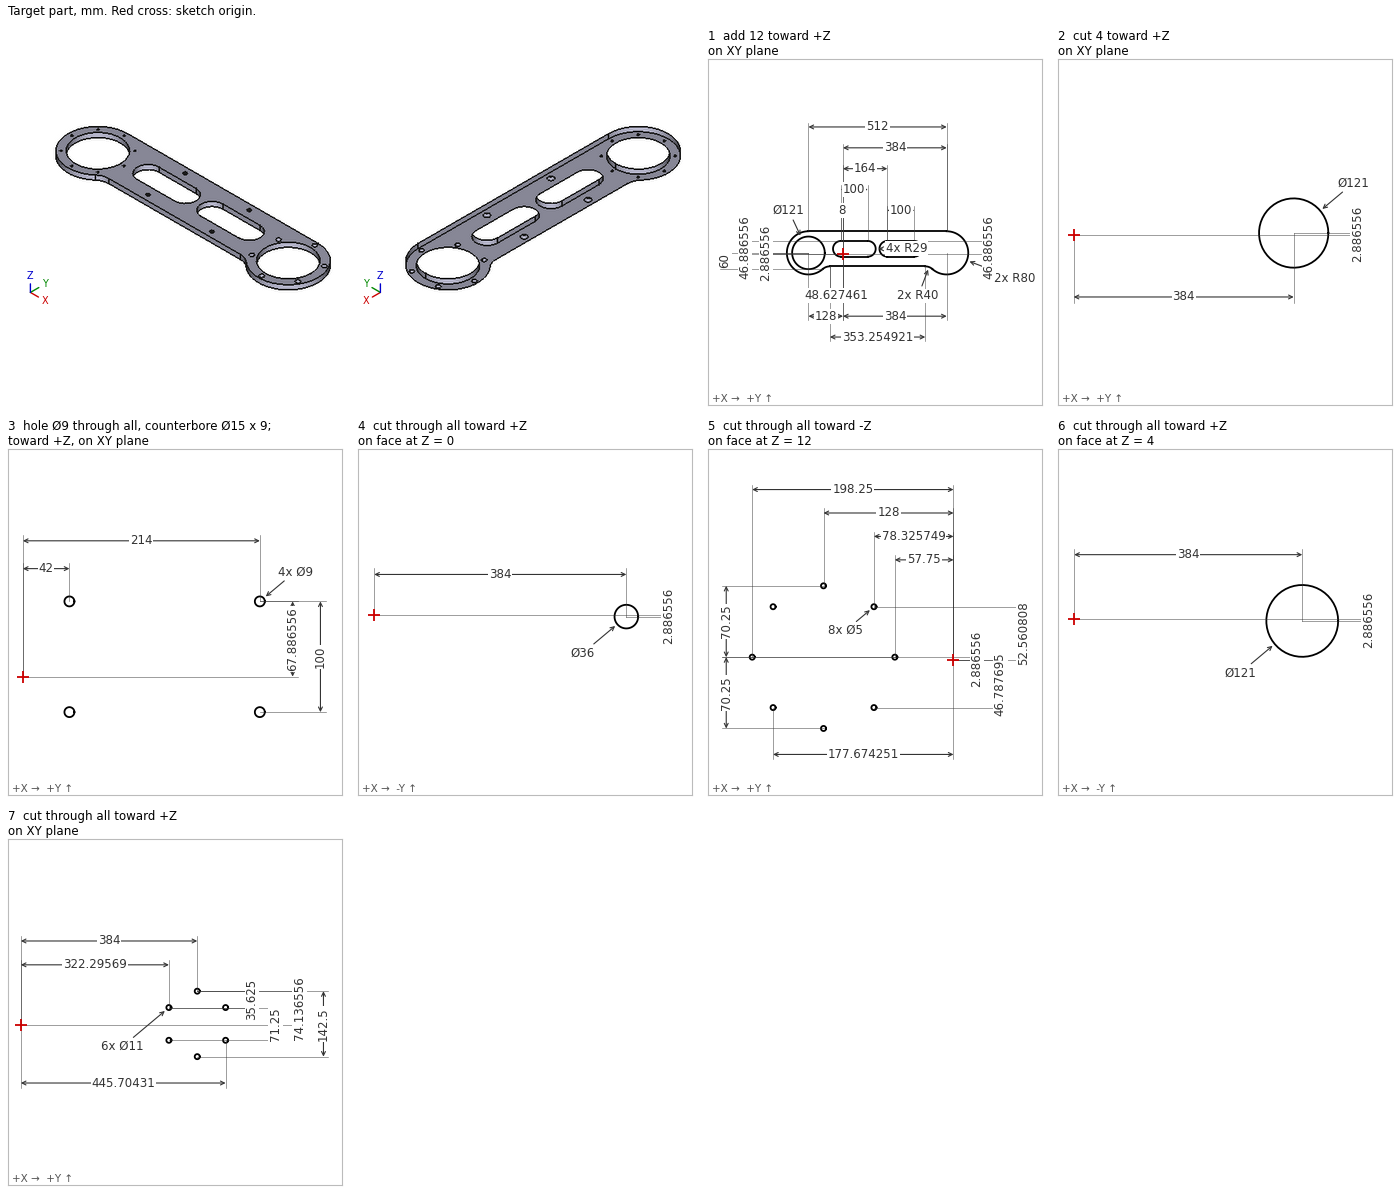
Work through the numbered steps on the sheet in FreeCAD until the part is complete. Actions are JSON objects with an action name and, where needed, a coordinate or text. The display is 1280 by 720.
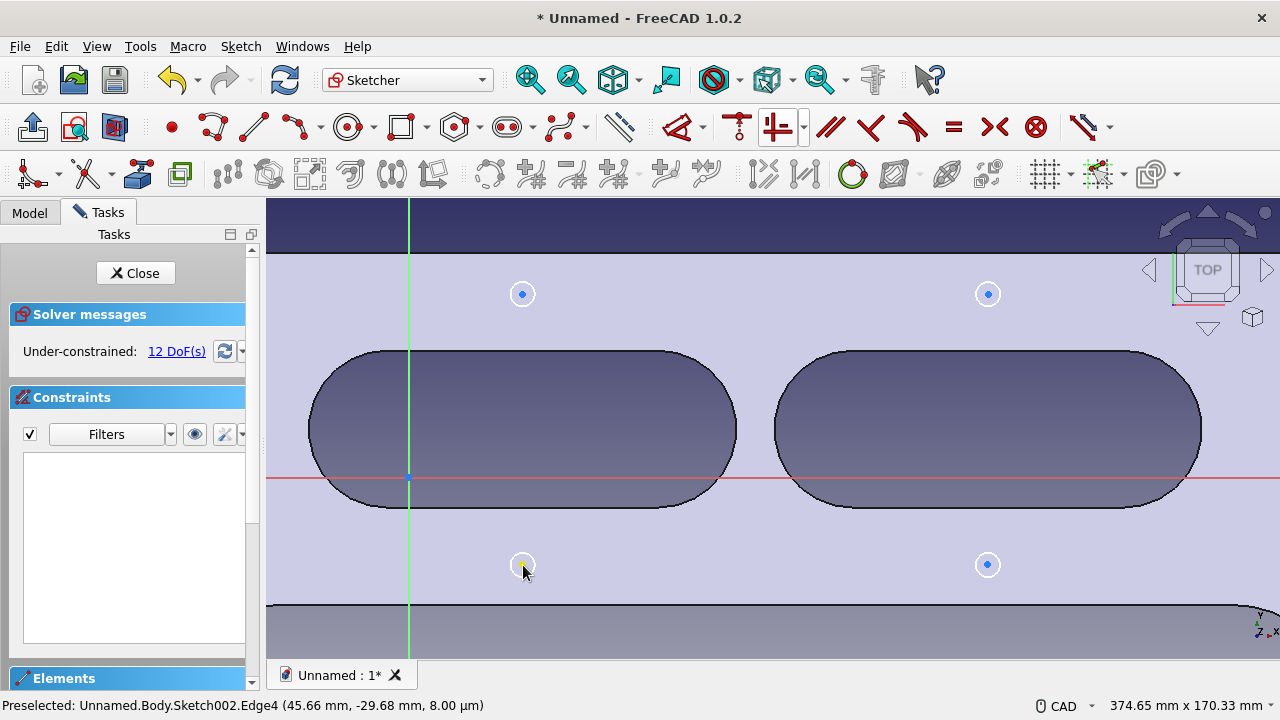
{"action": "left_click", "coordinate": [997, 286]}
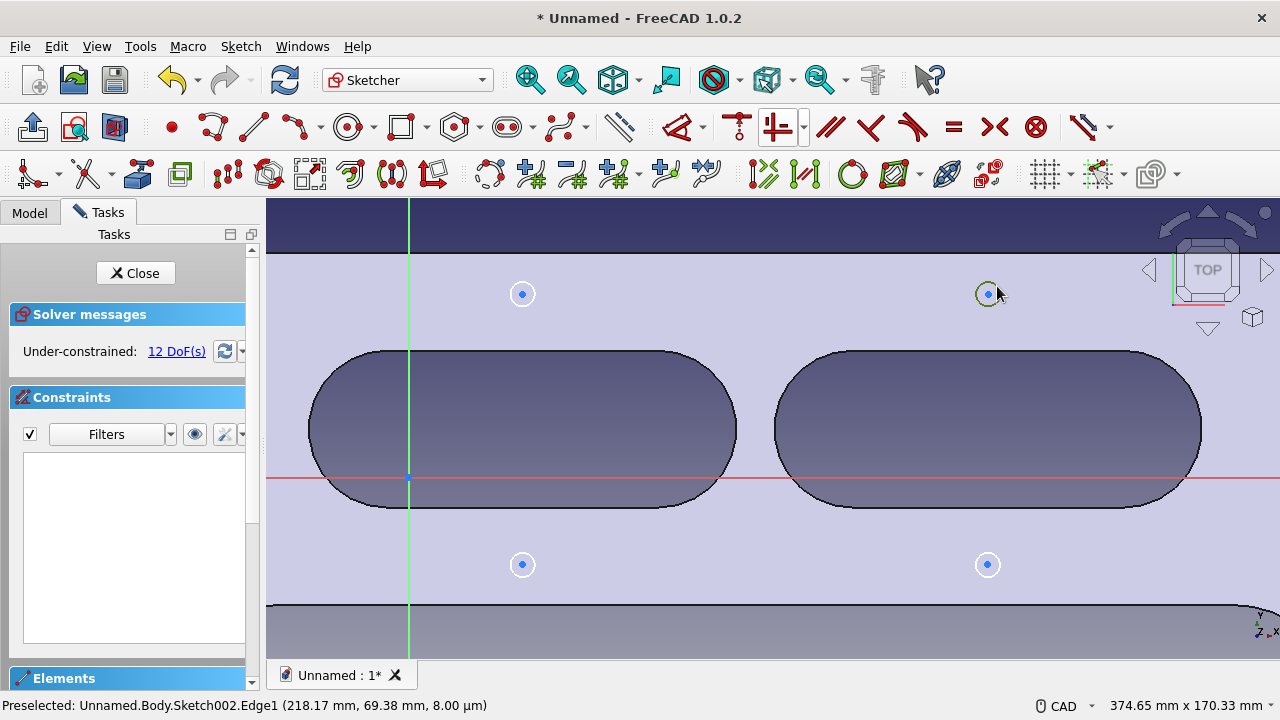
{"action": "left_click", "coordinate": [996, 556]}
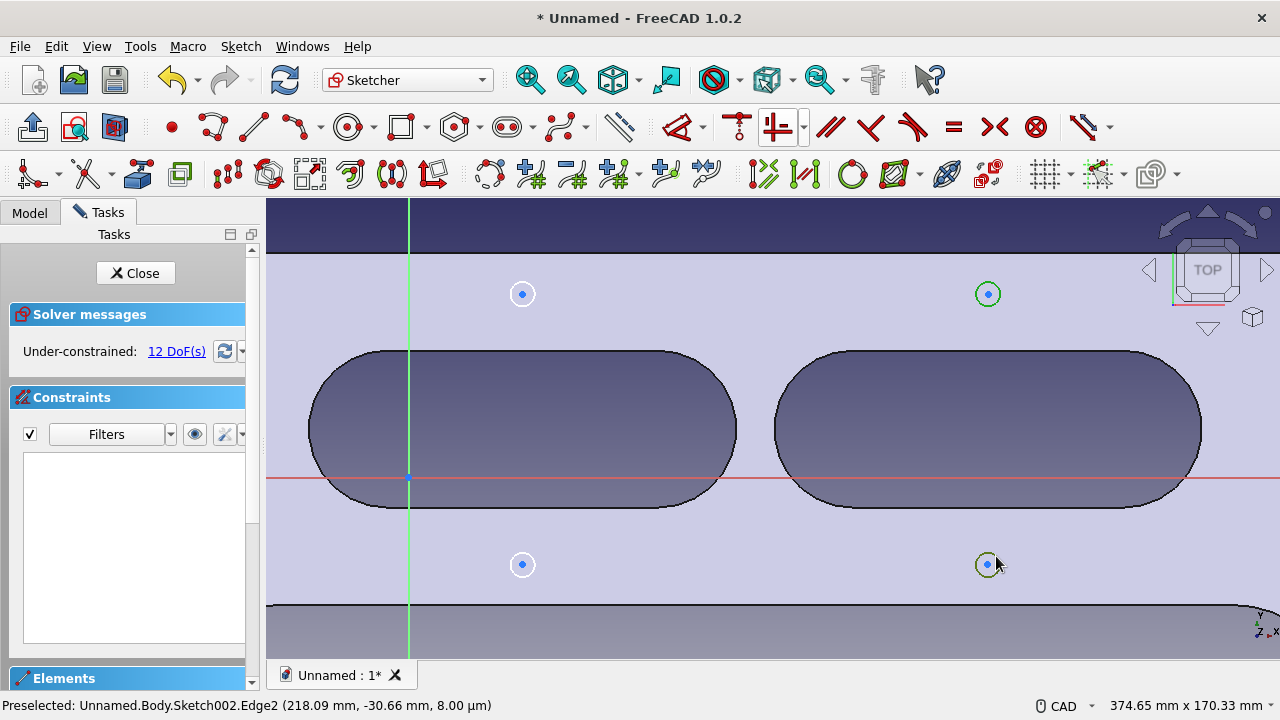
{"action": "left_click", "coordinate": [531, 286]}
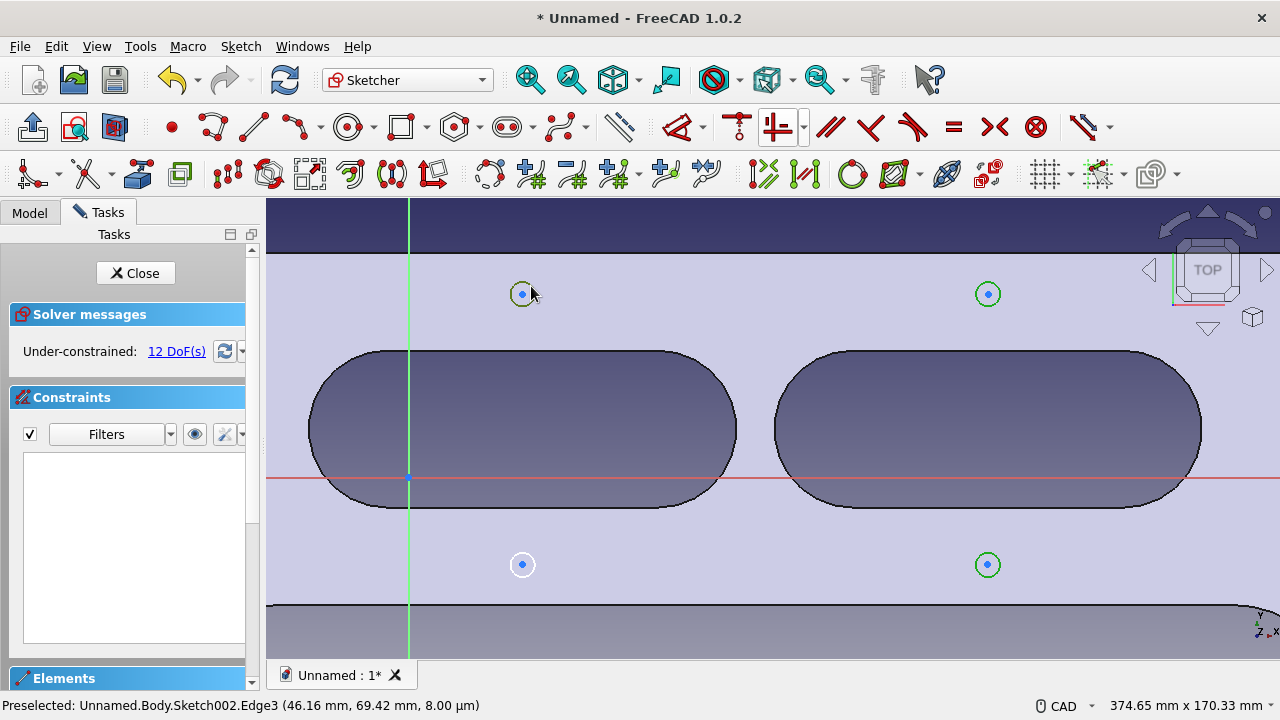
{"action": "left_click", "coordinate": [531, 556]}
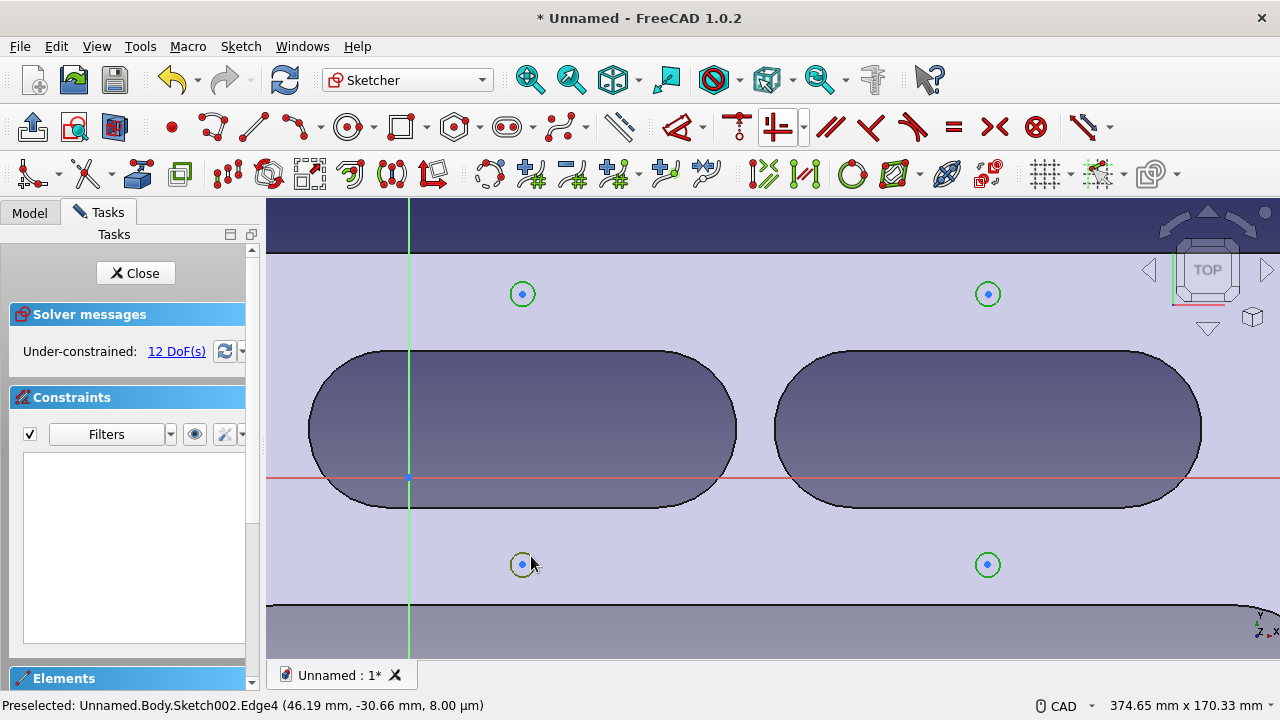
{"action": "left_click", "coordinate": [954, 128]}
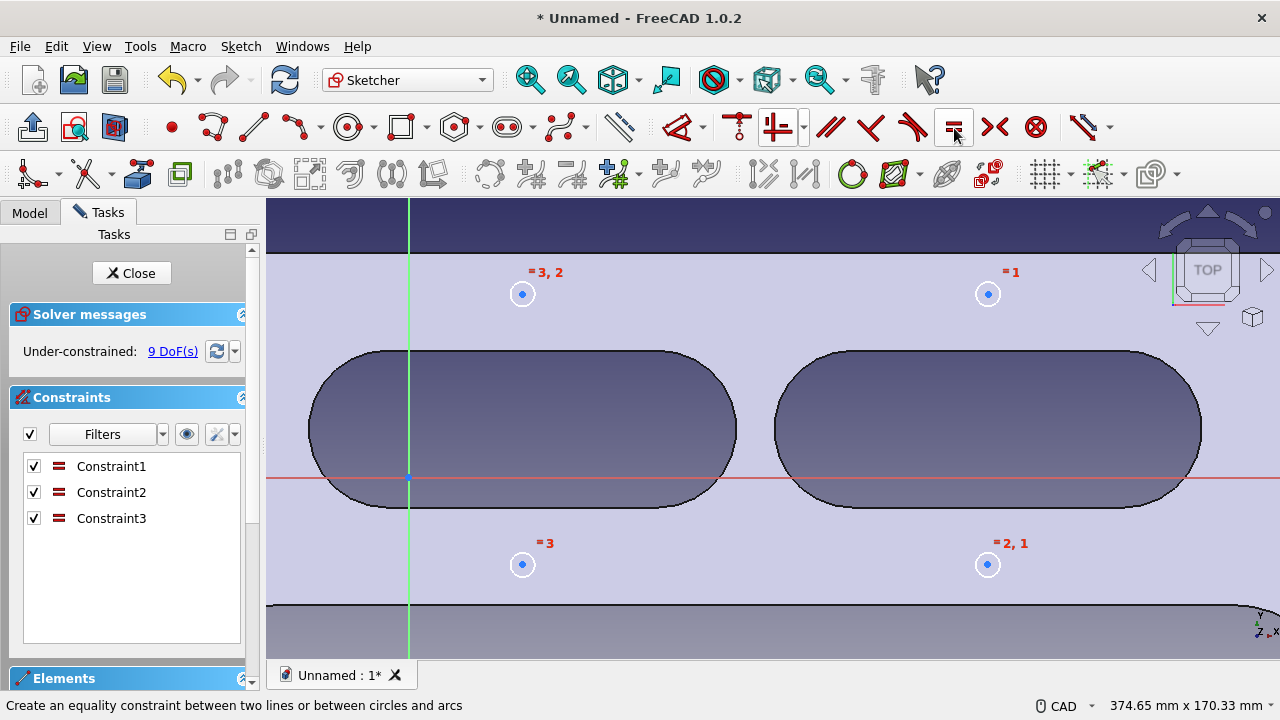
{"action": "left_click", "coordinate": [988, 294]}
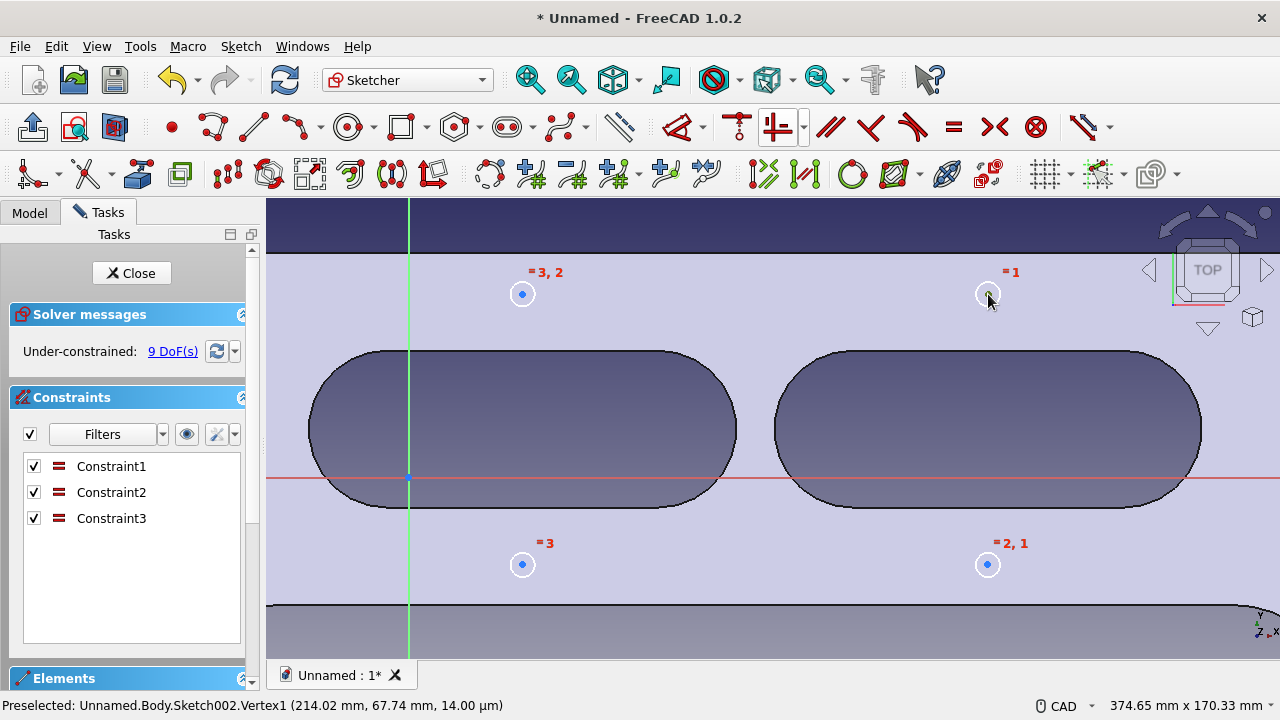
{"action": "left_click", "coordinate": [988, 565]}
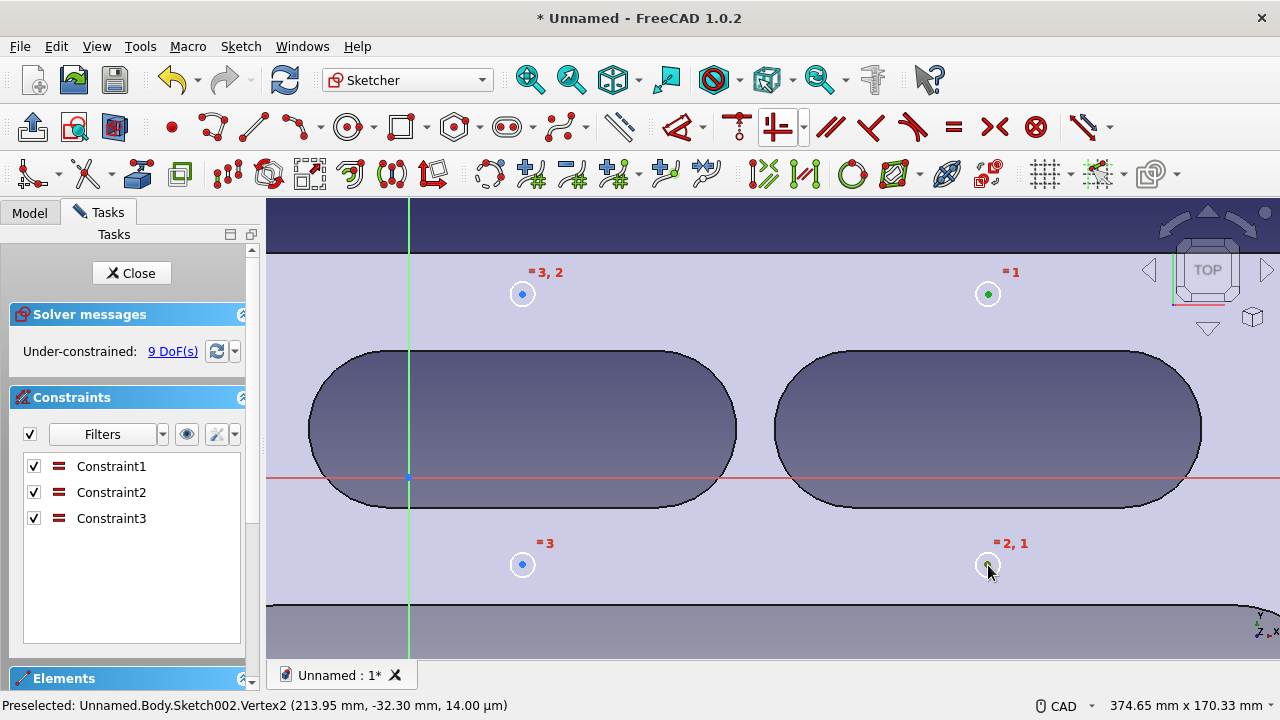
{"action": "key", "text": "v"}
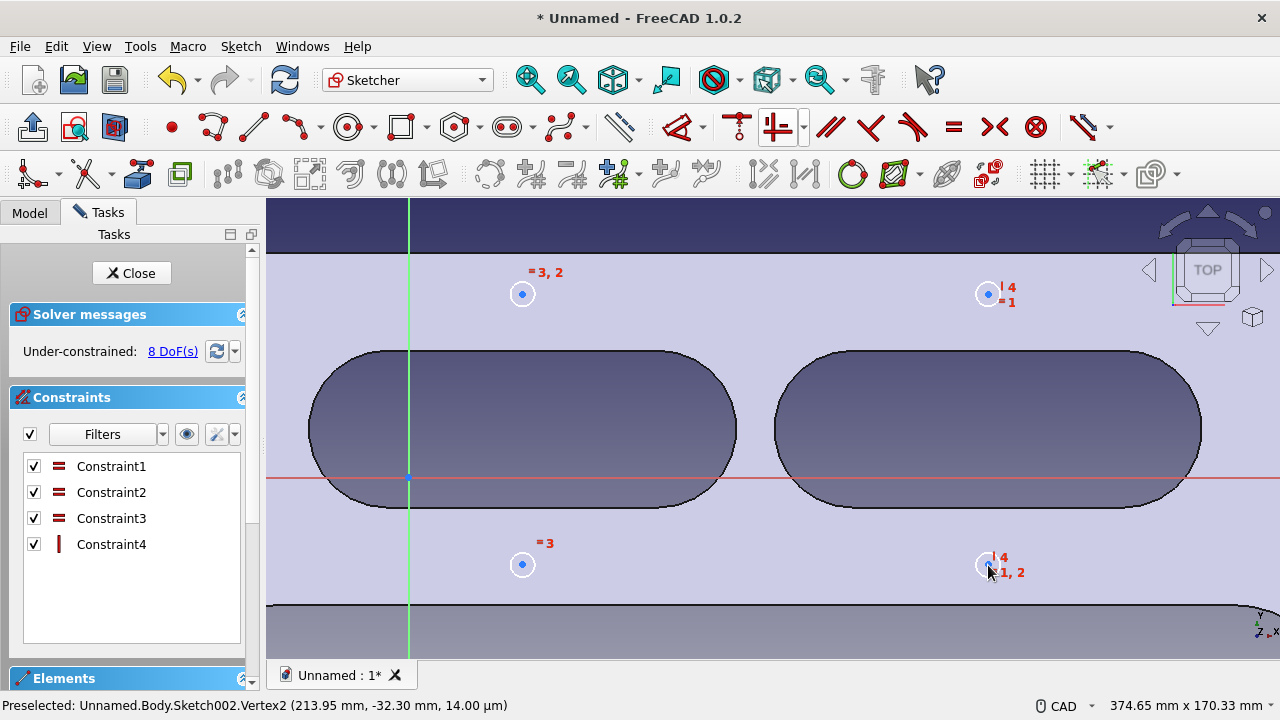
{"action": "left_click", "coordinate": [988, 294]}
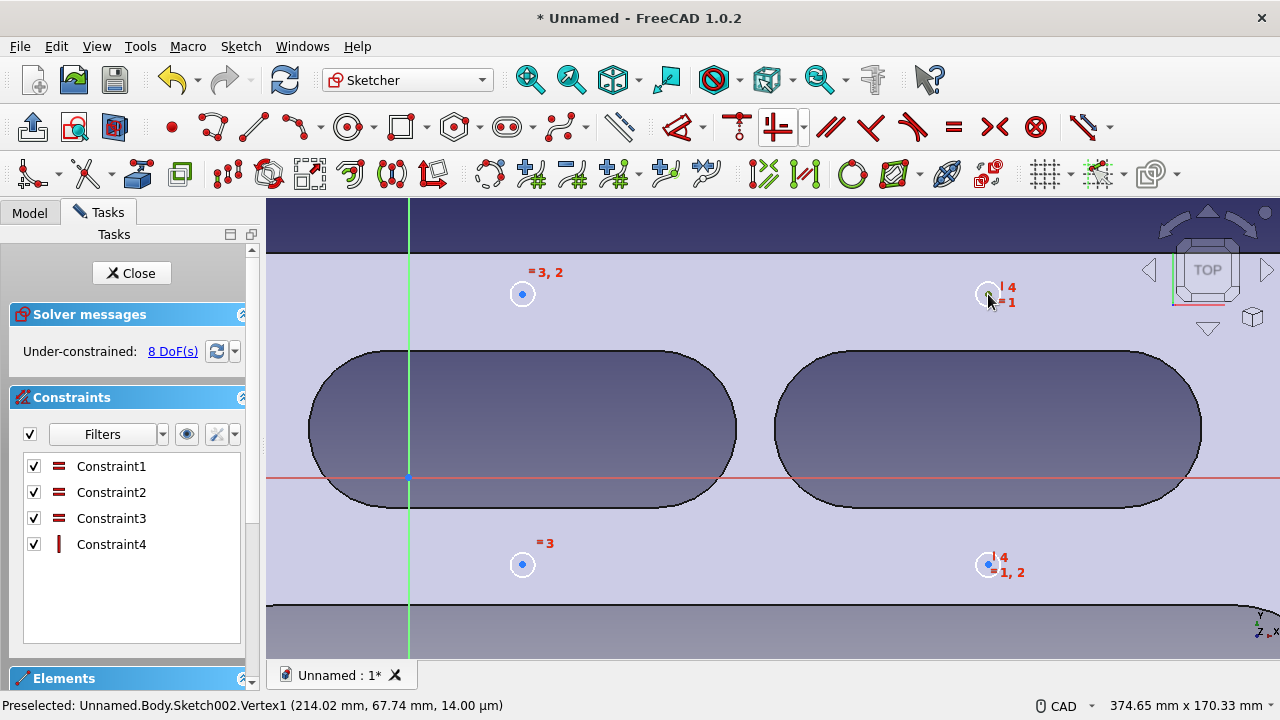
{"action": "left_click", "coordinate": [523, 294]}